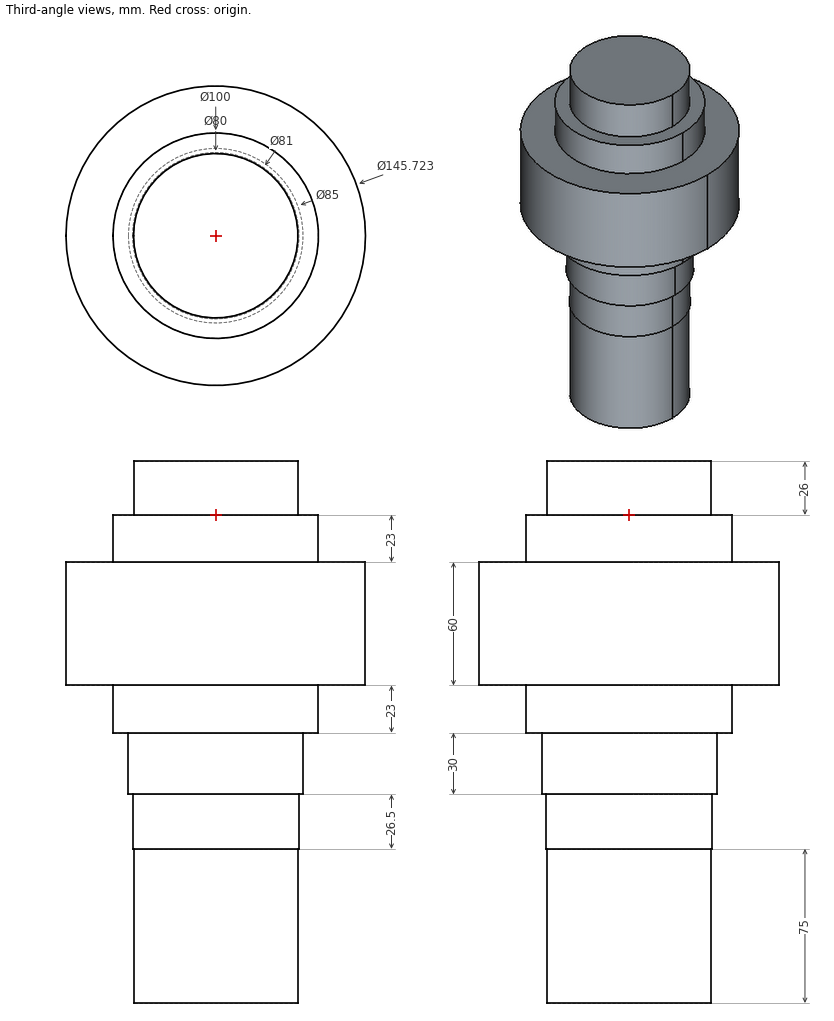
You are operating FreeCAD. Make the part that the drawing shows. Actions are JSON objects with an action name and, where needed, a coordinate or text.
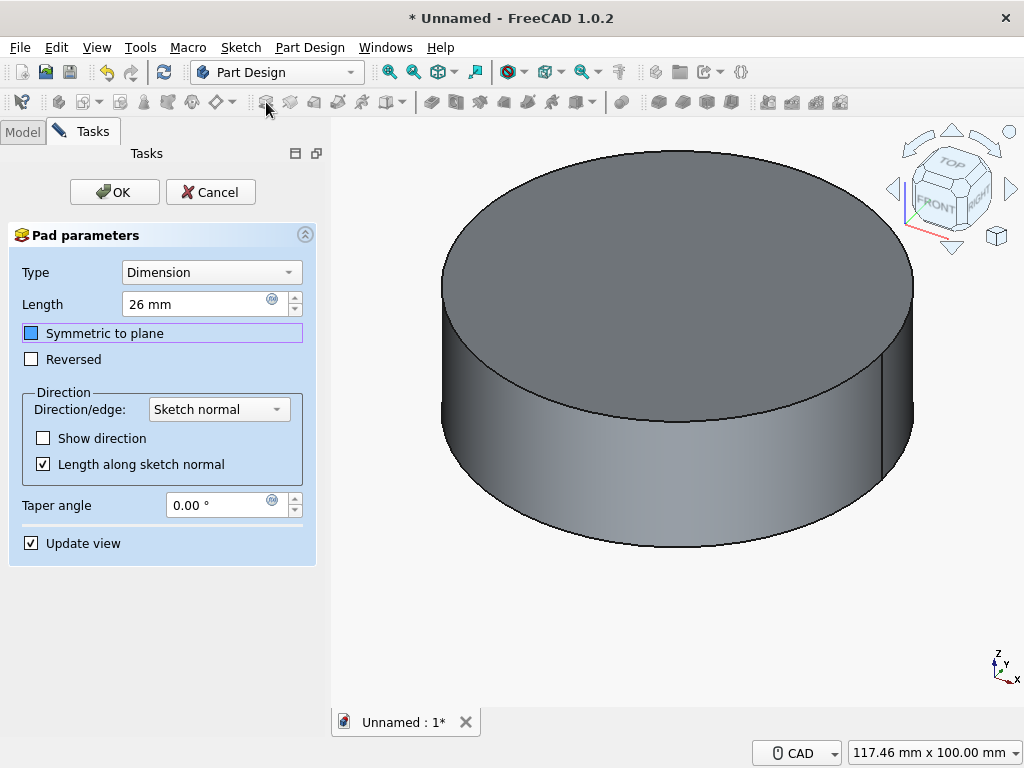
{"action": "left_click", "coordinate": [115, 192]}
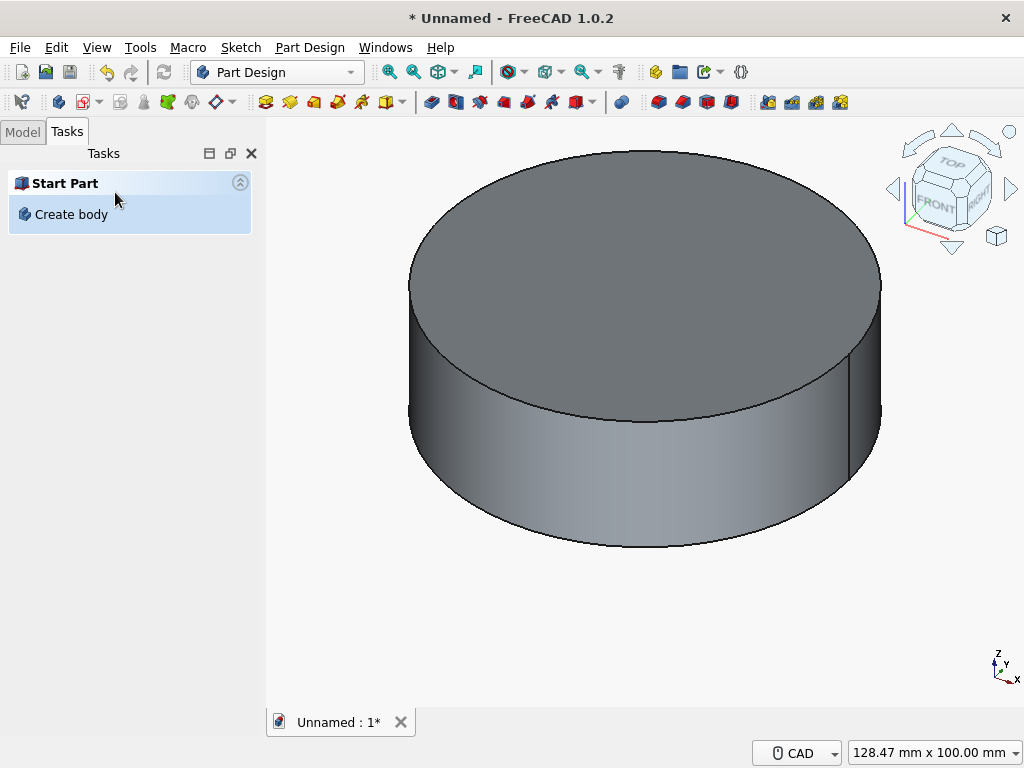
{"action": "key", "text": "v f"}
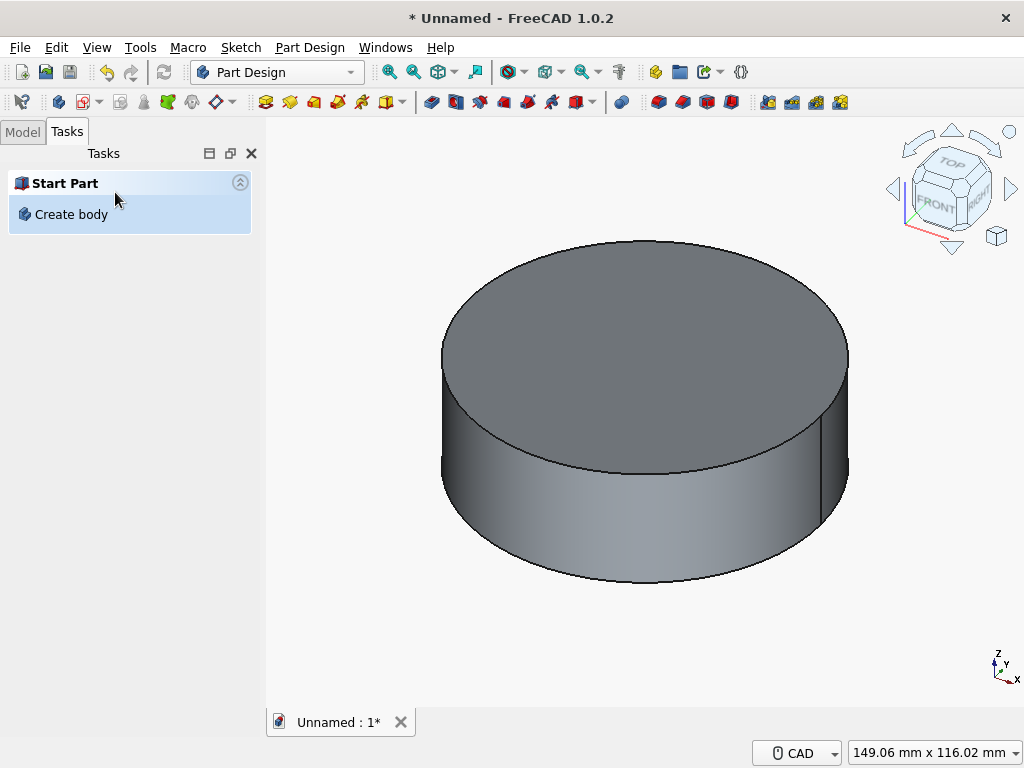
{"action": "key", "text": "5"}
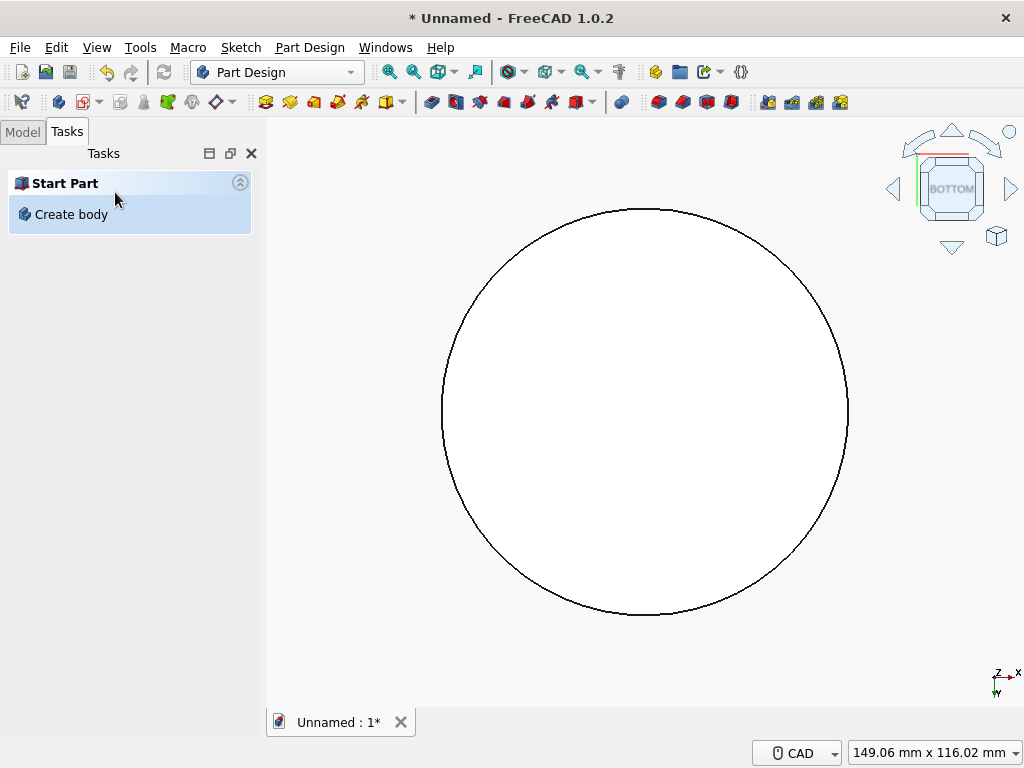
{"action": "left_click", "coordinate": [645, 411]}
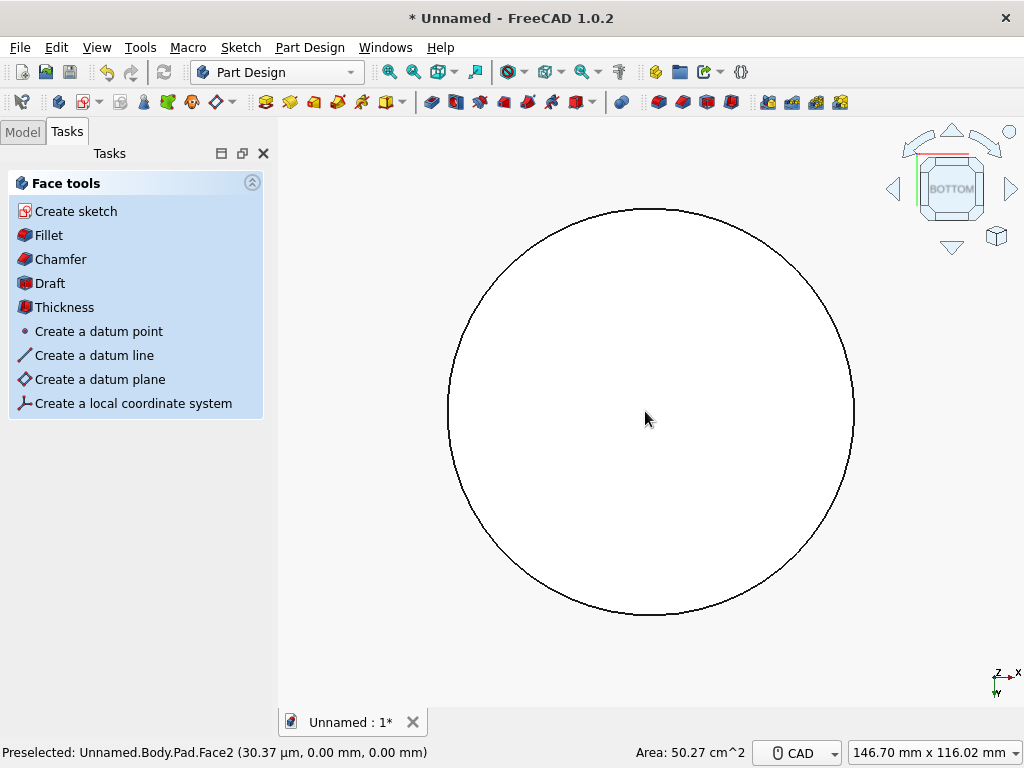
{"action": "left_click", "coordinate": [84, 102]}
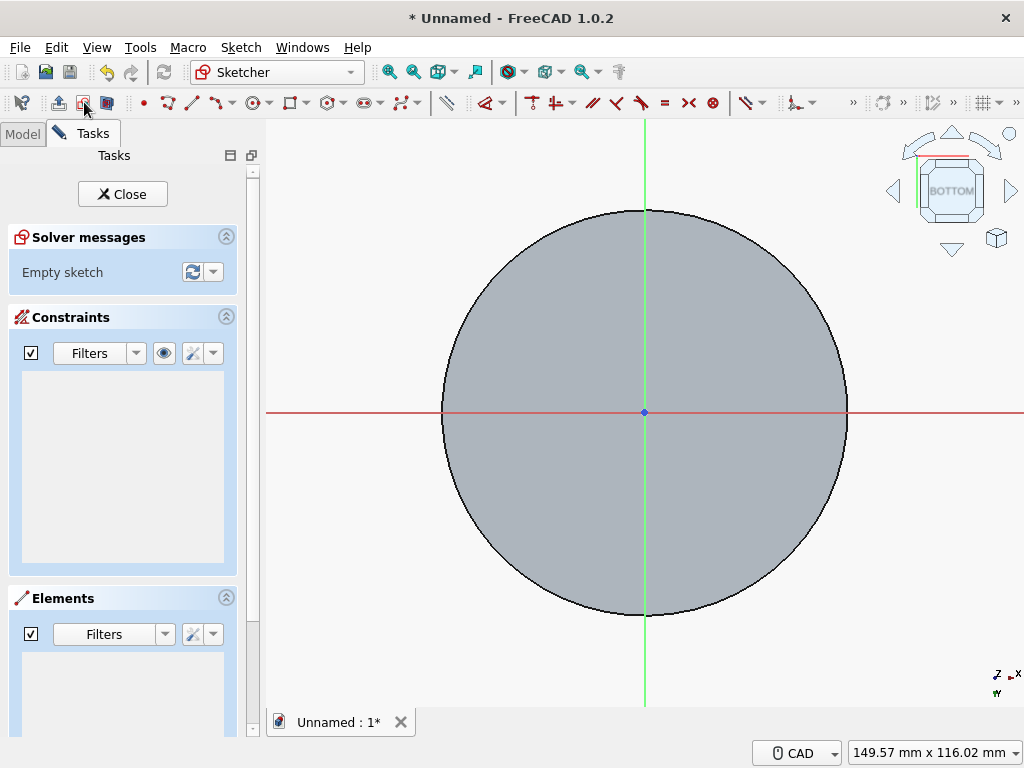
{"action": "scroll", "coordinate": [294, 413], "scroll_direction": "down", "scroll_amount": 1}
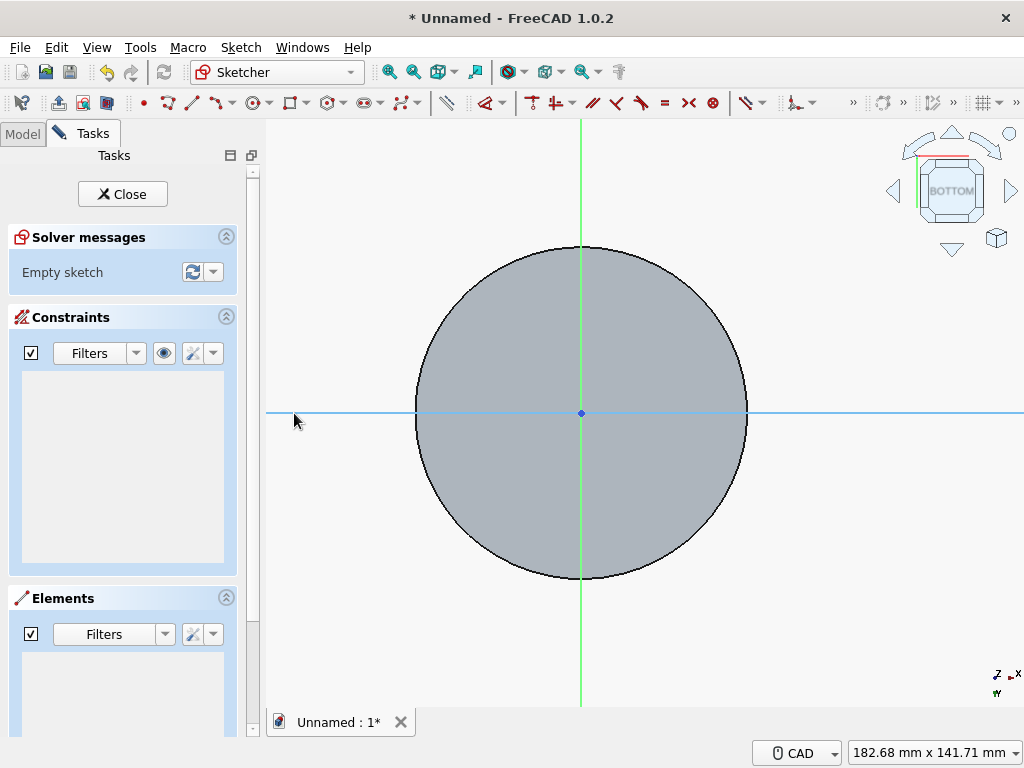
{"action": "left_click", "coordinate": [254, 104]}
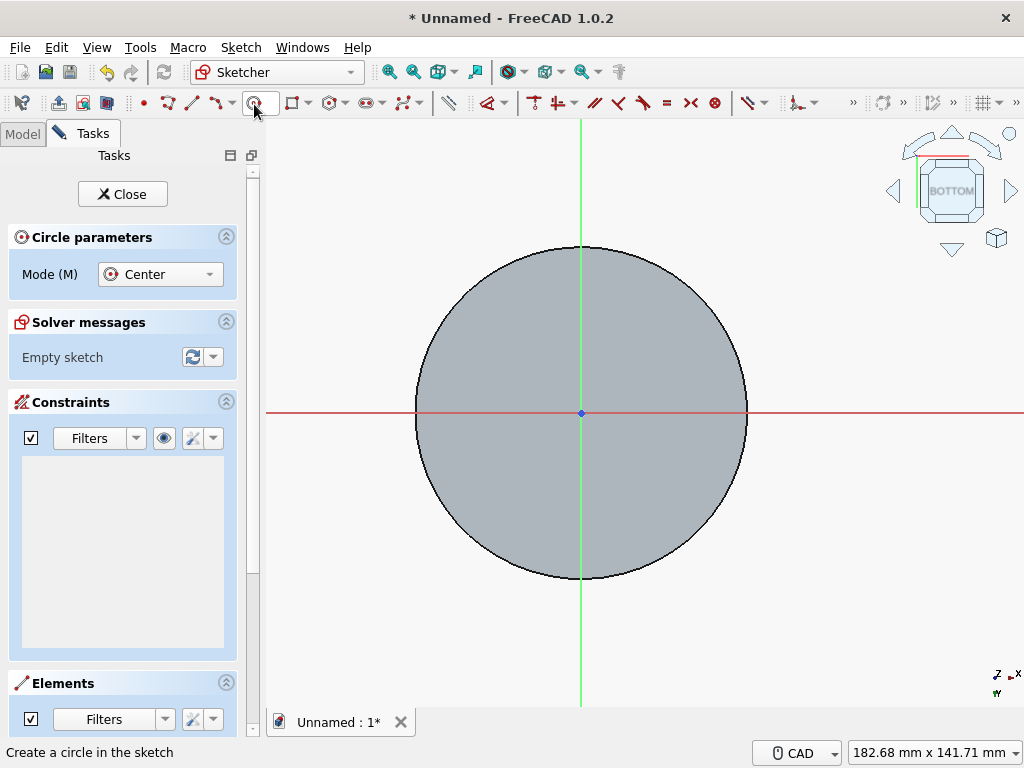
{"action": "left_click", "coordinate": [581, 413]}
{"action": "left_click", "coordinate": [728, 266]}
{"action": "key", "text": "Escape"}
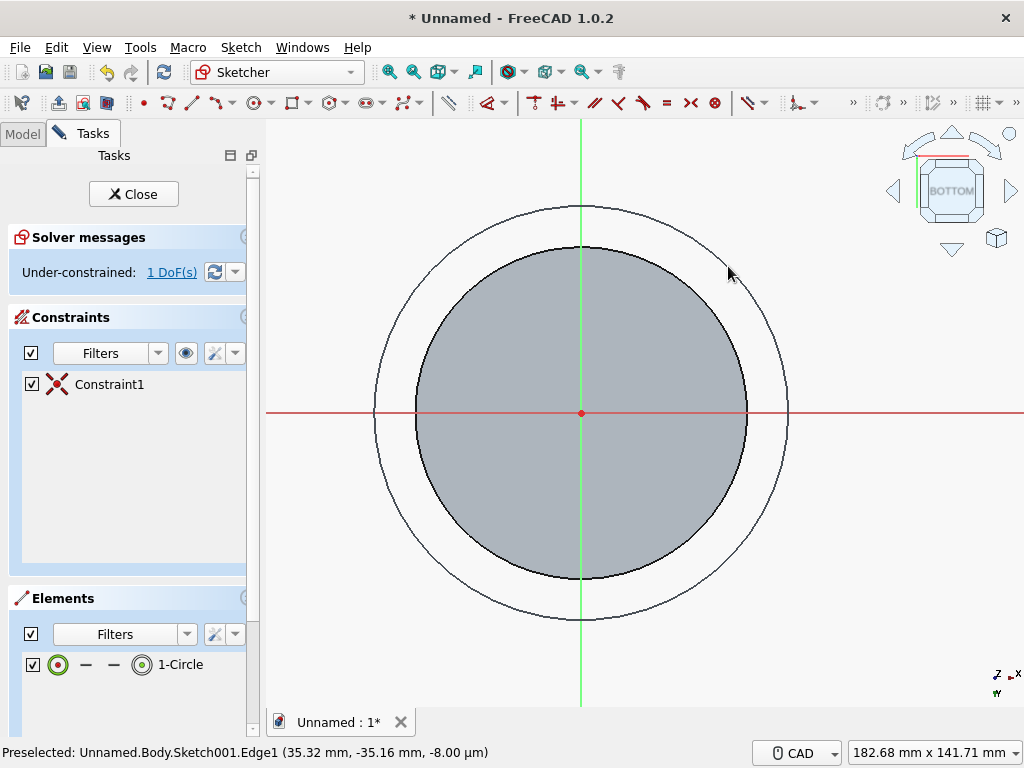
{"action": "key", "text": "d"}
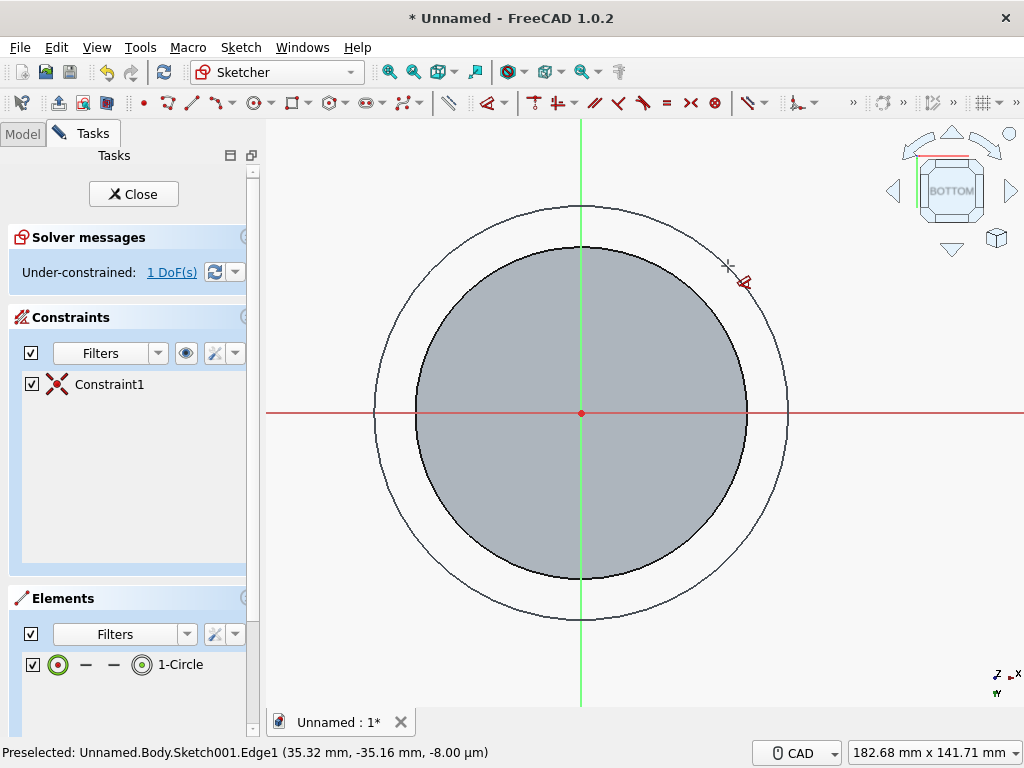
{"action": "left_click", "coordinate": [727, 266]}
{"action": "left_click", "coordinate": [750, 243]}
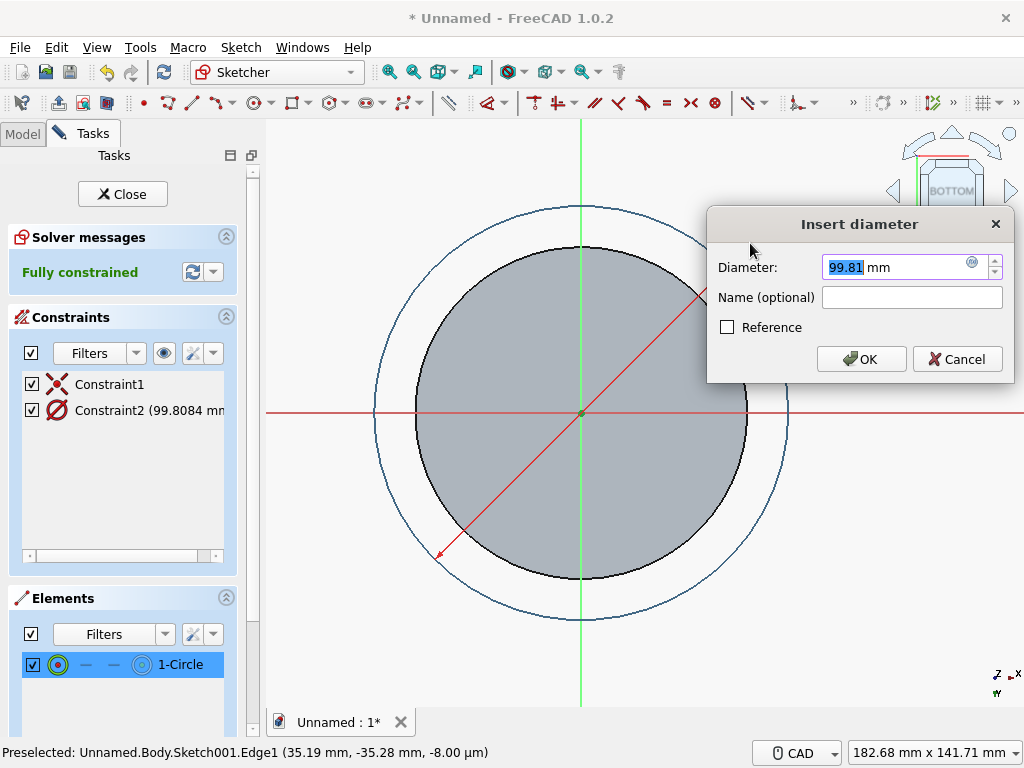
{"action": "type", "text": "100"}
{"action": "key", "text": "Return"}
{"action": "key", "text": "Escape"}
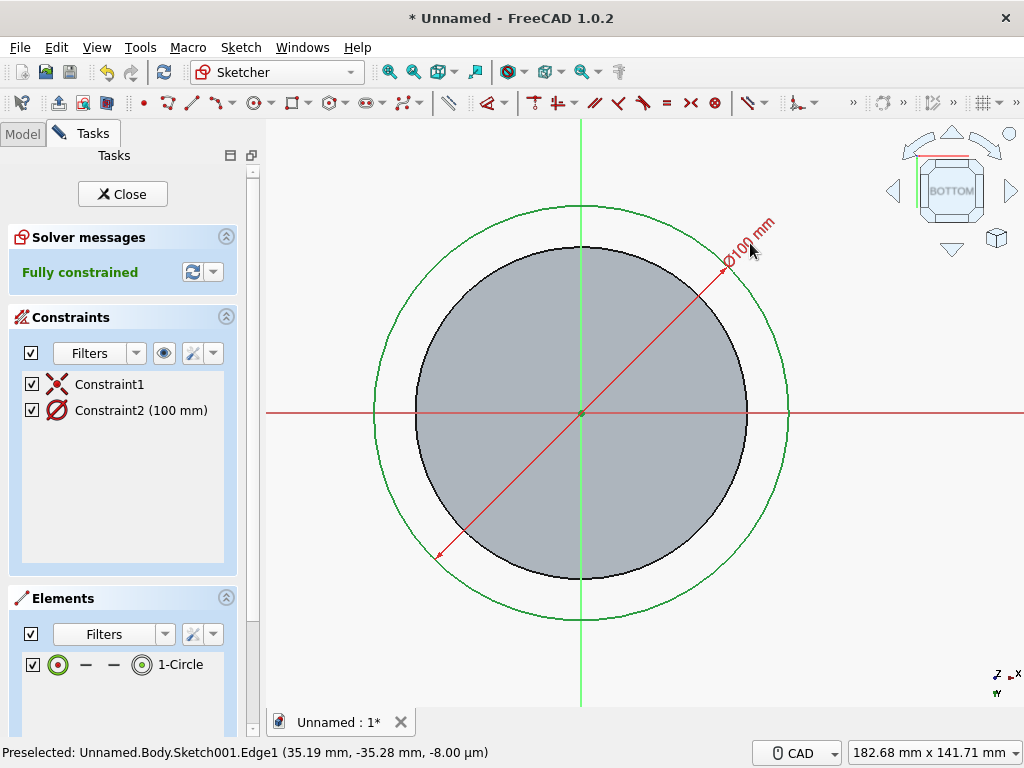
{"action": "left_click", "coordinate": [123, 194]}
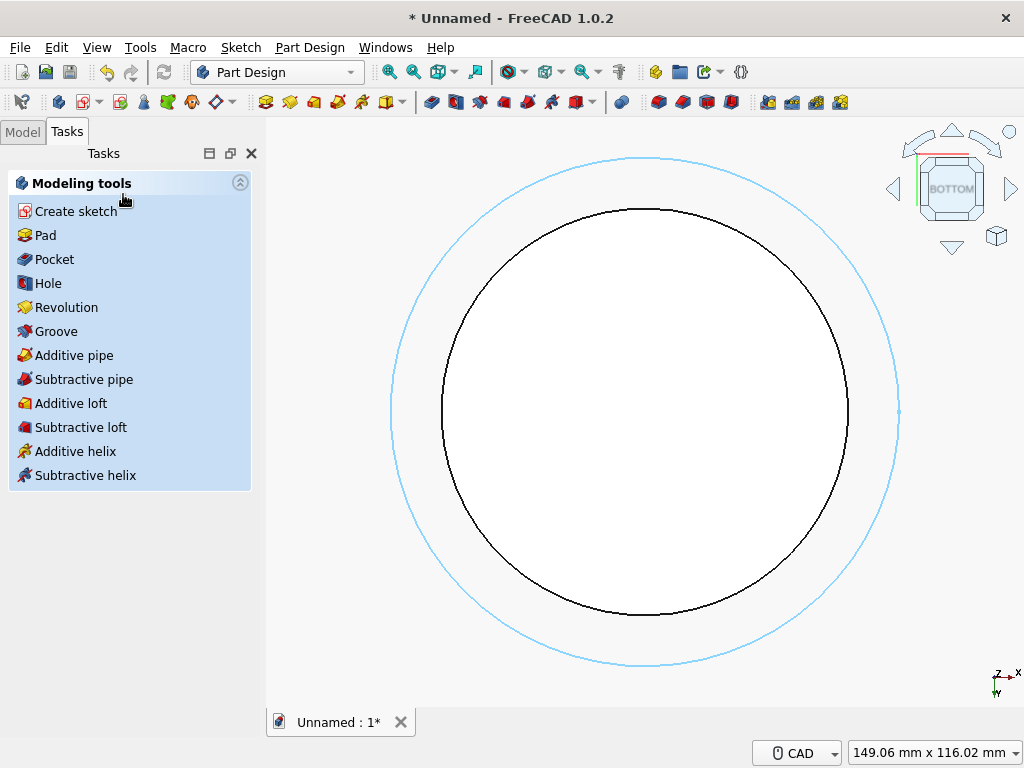
{"action": "left_click", "coordinate": [266, 102]}